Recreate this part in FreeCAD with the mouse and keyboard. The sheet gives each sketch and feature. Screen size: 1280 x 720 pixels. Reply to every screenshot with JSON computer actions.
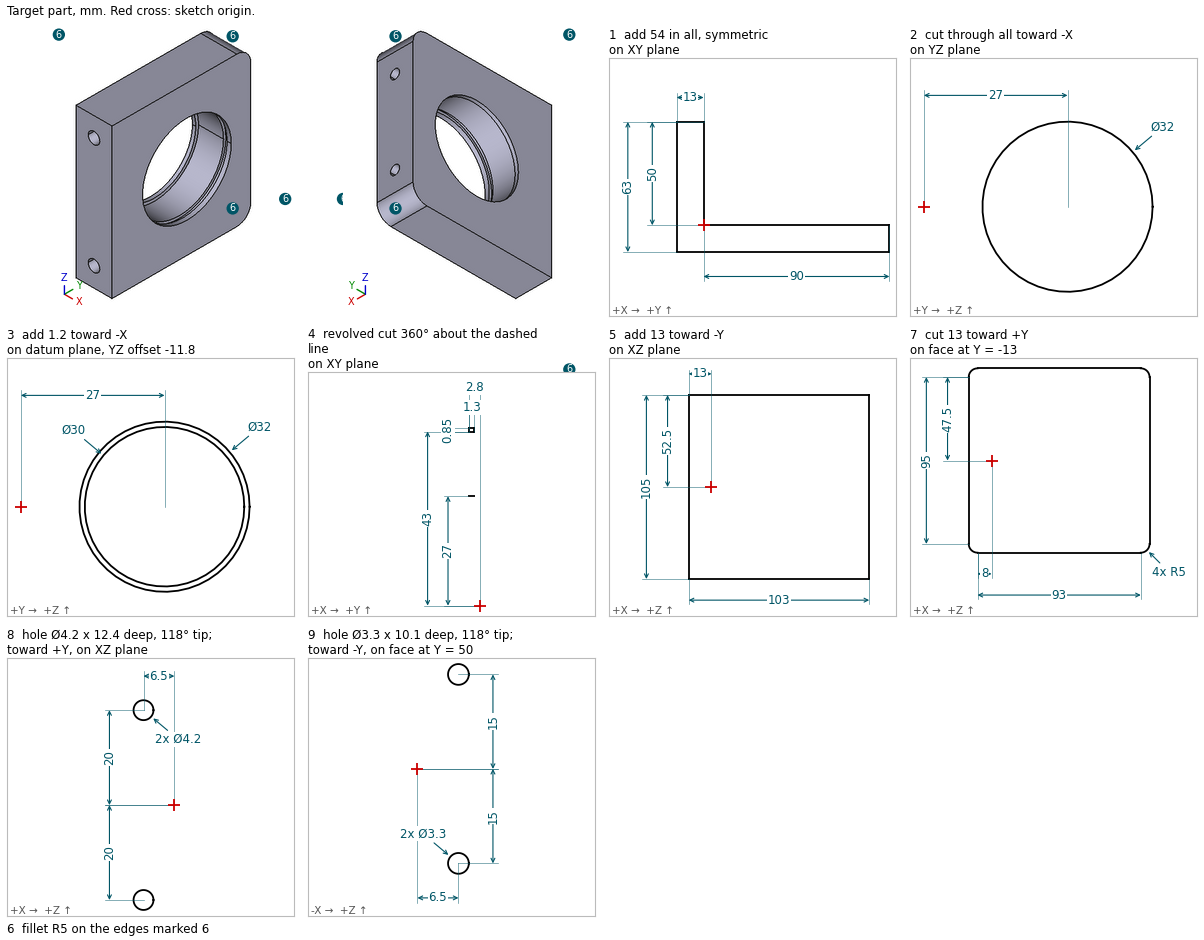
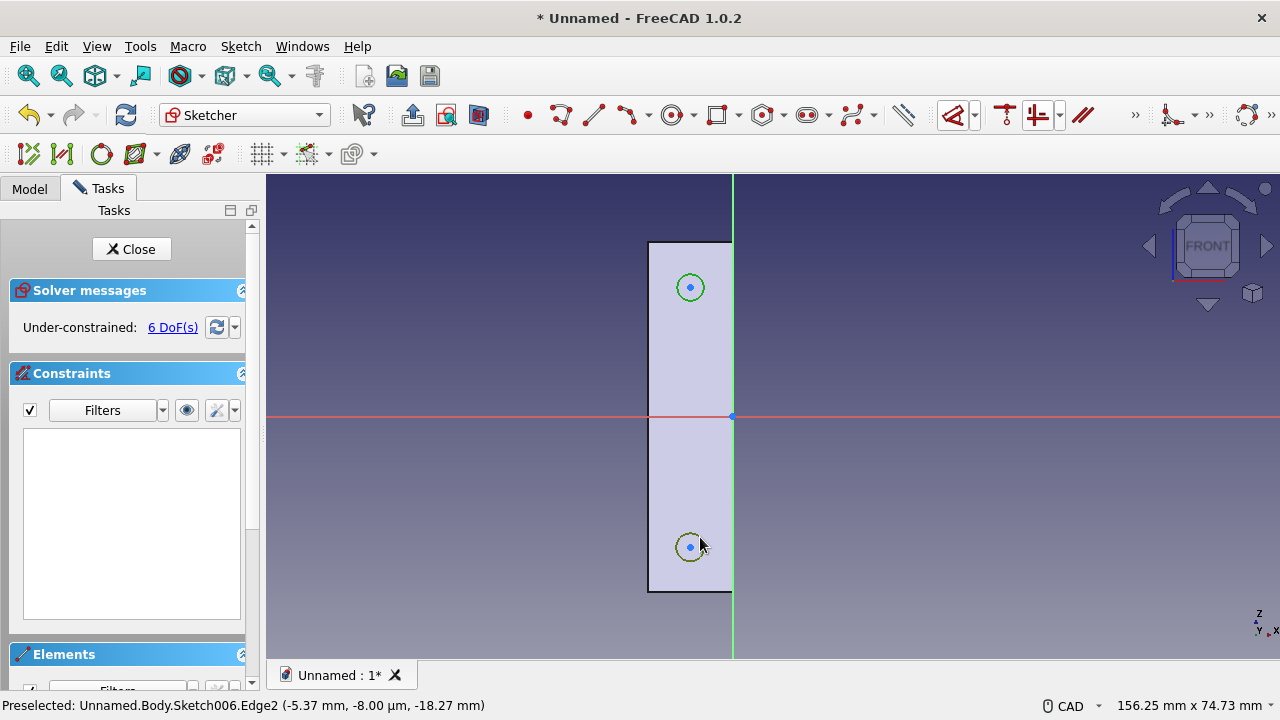
{"action": "key", "text": "e"}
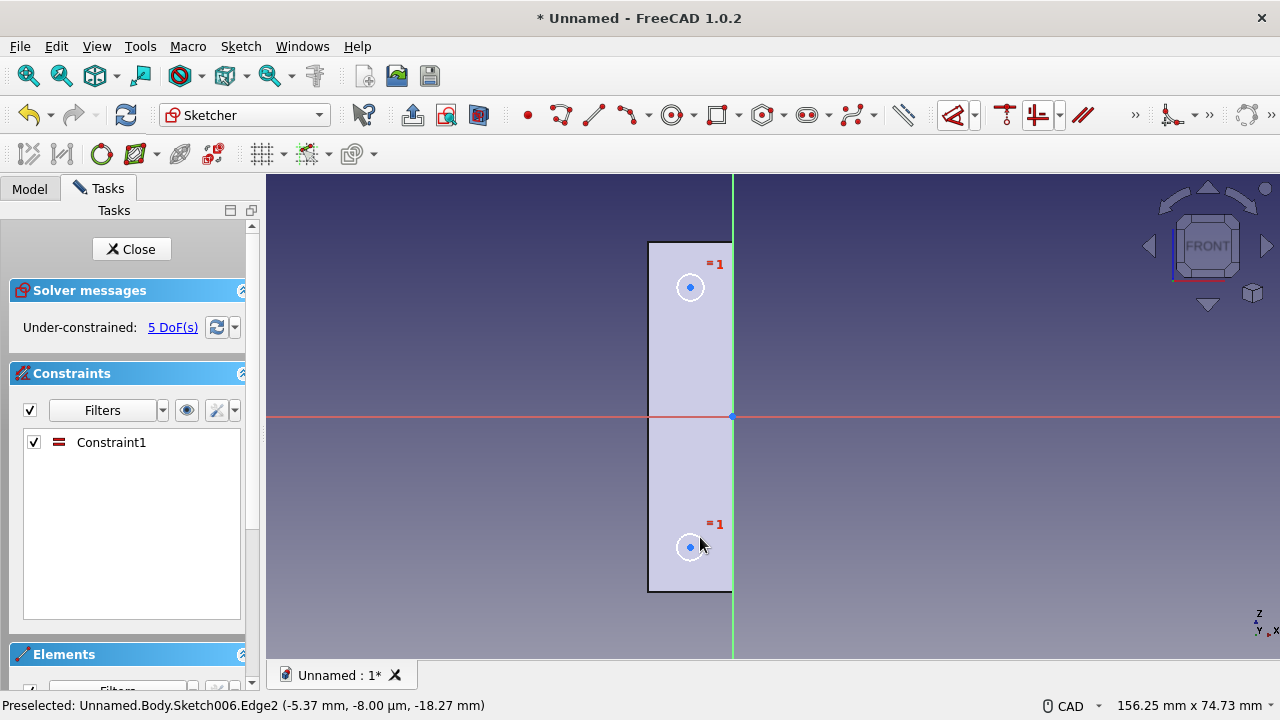
{"action": "left_click", "coordinate": [691, 288]}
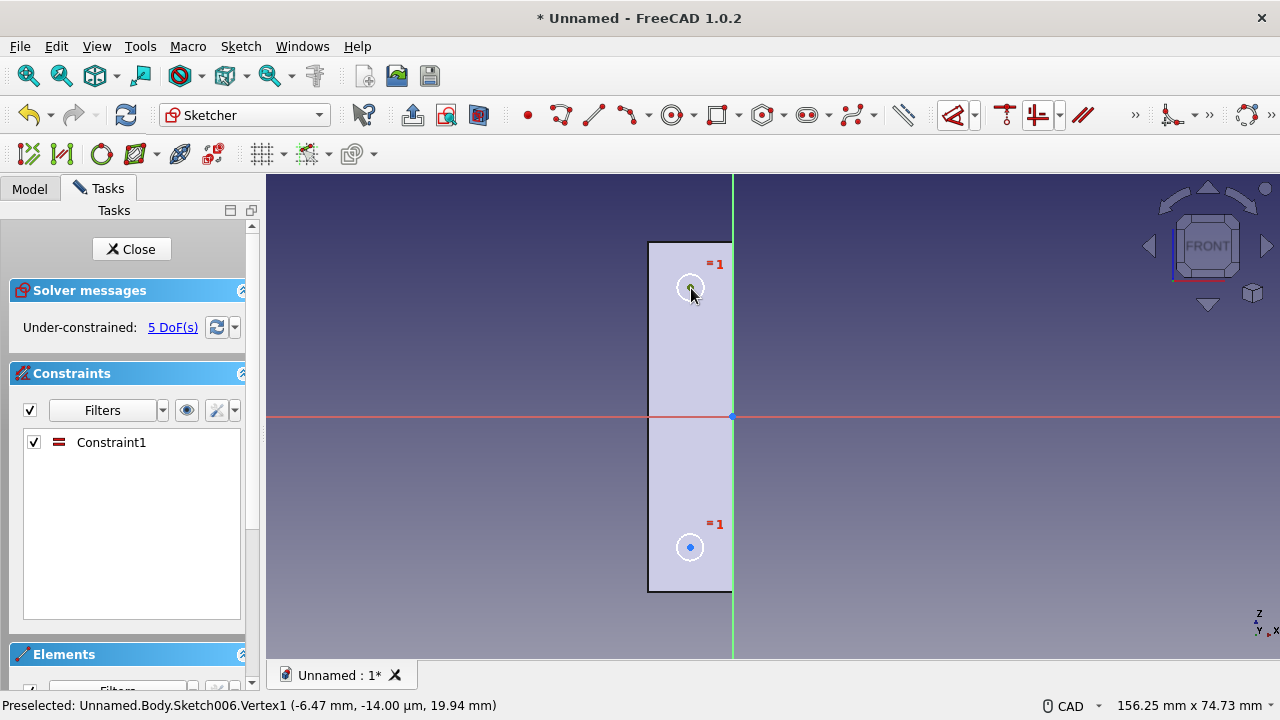
{"action": "left_click", "coordinate": [690, 547]}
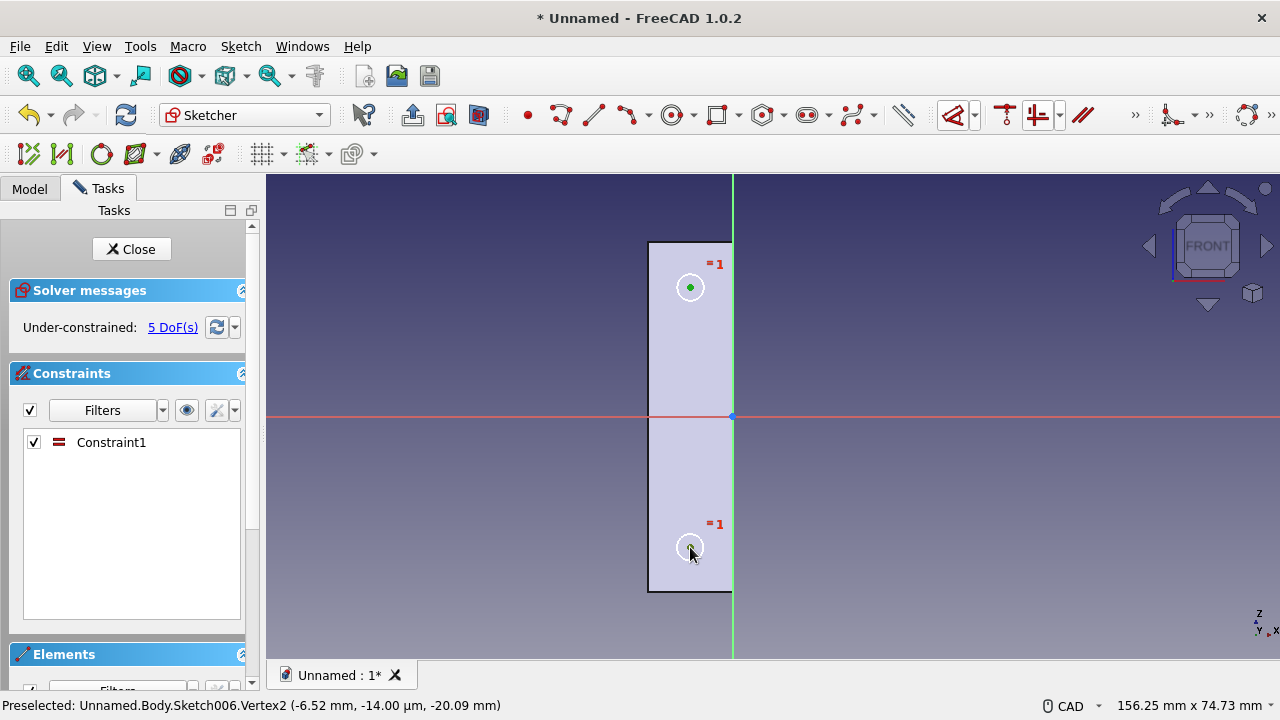
{"action": "key", "text": "v"}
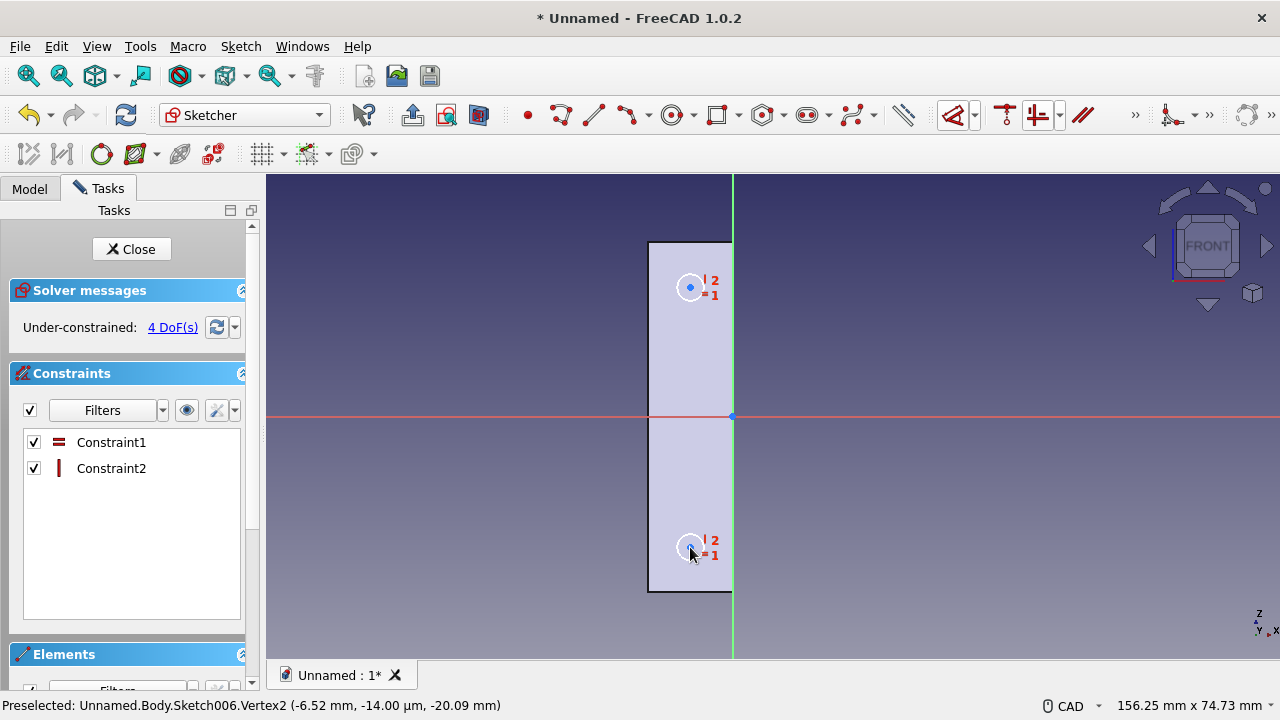
{"action": "scroll", "coordinate": [700, 278], "scroll_direction": "up", "scroll_amount": 2}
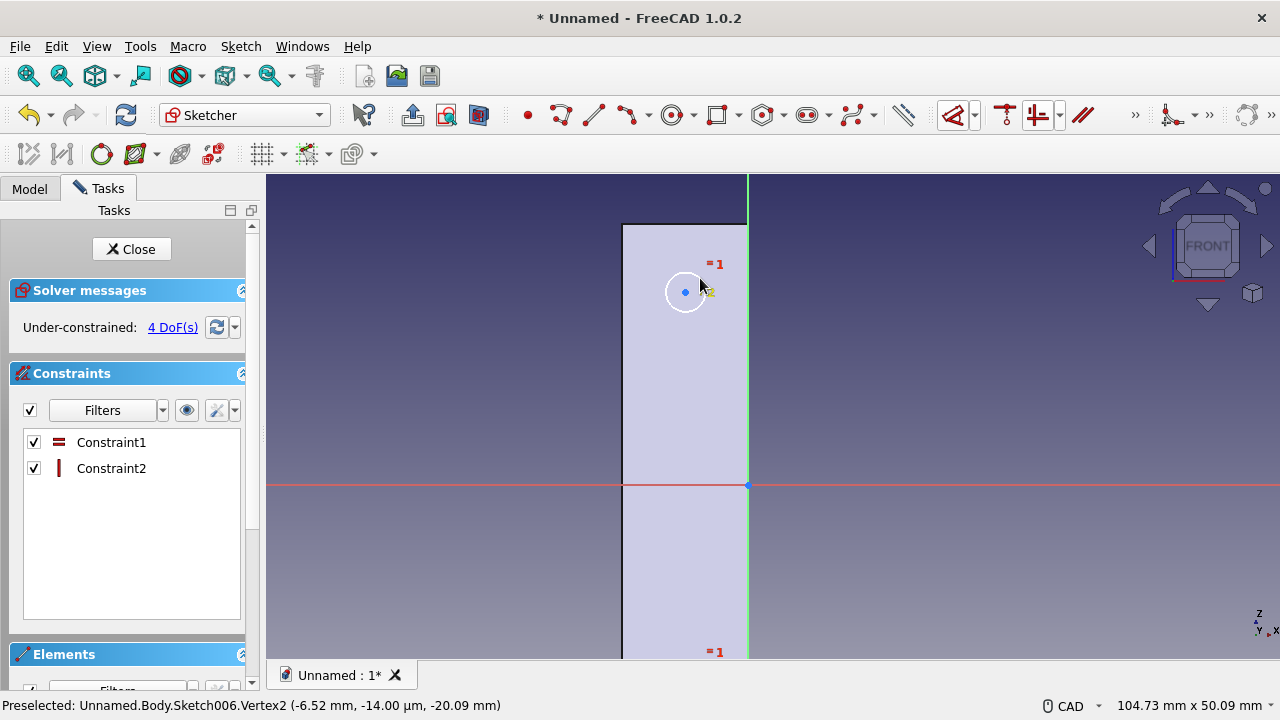
{"action": "left_click", "coordinate": [700, 278]}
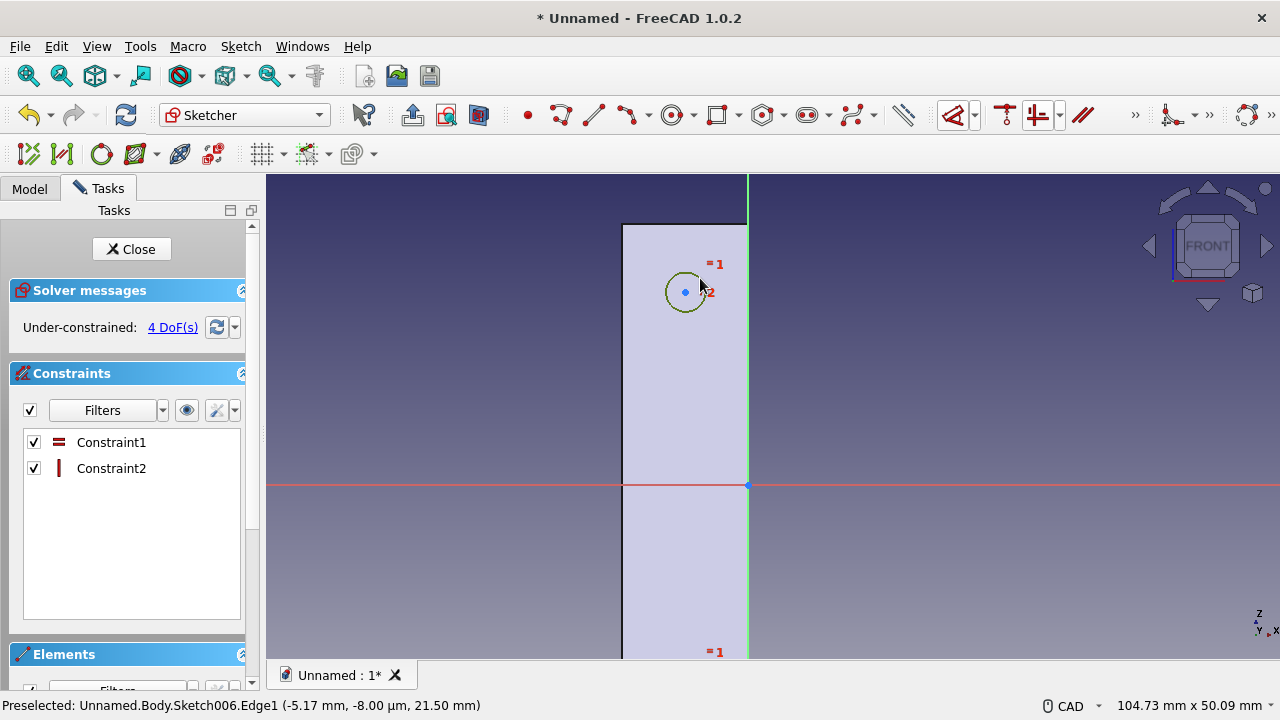
{"action": "left_click", "coordinate": [974, 116]}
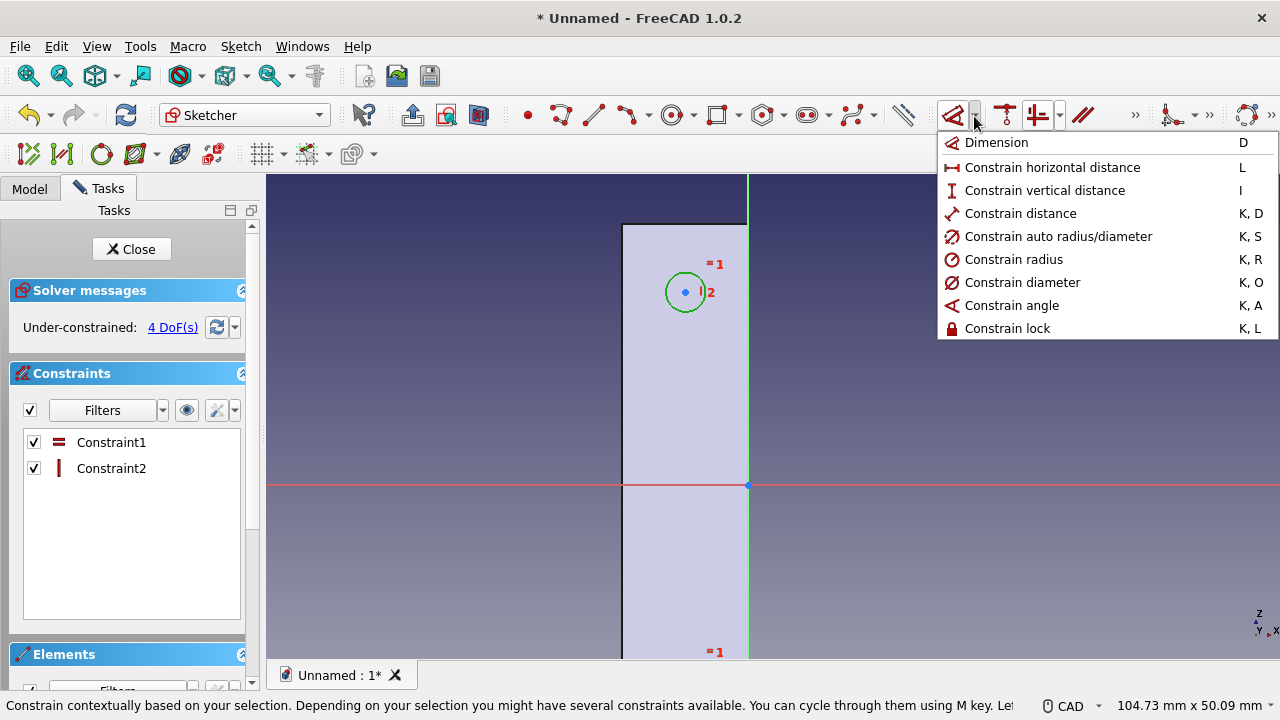
{"action": "left_click", "coordinate": [1108, 282]}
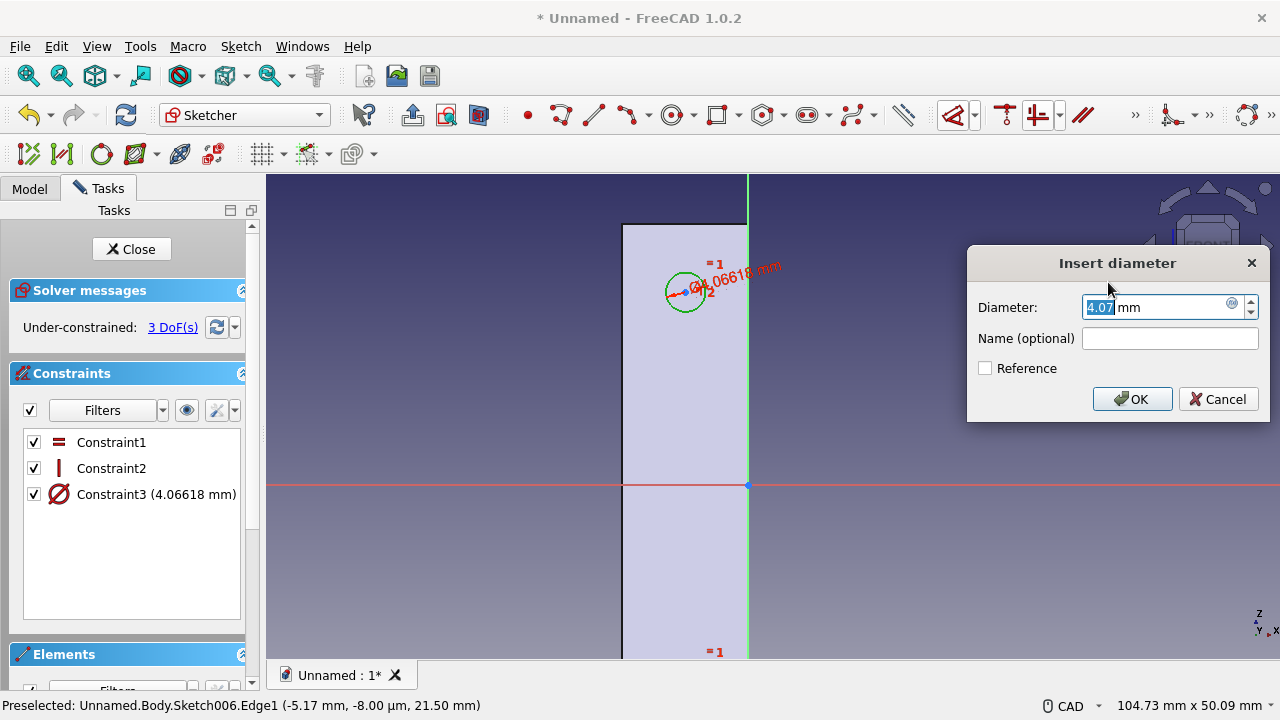
{"action": "type", "text": "4.2"}
{"action": "key", "text": "Return"}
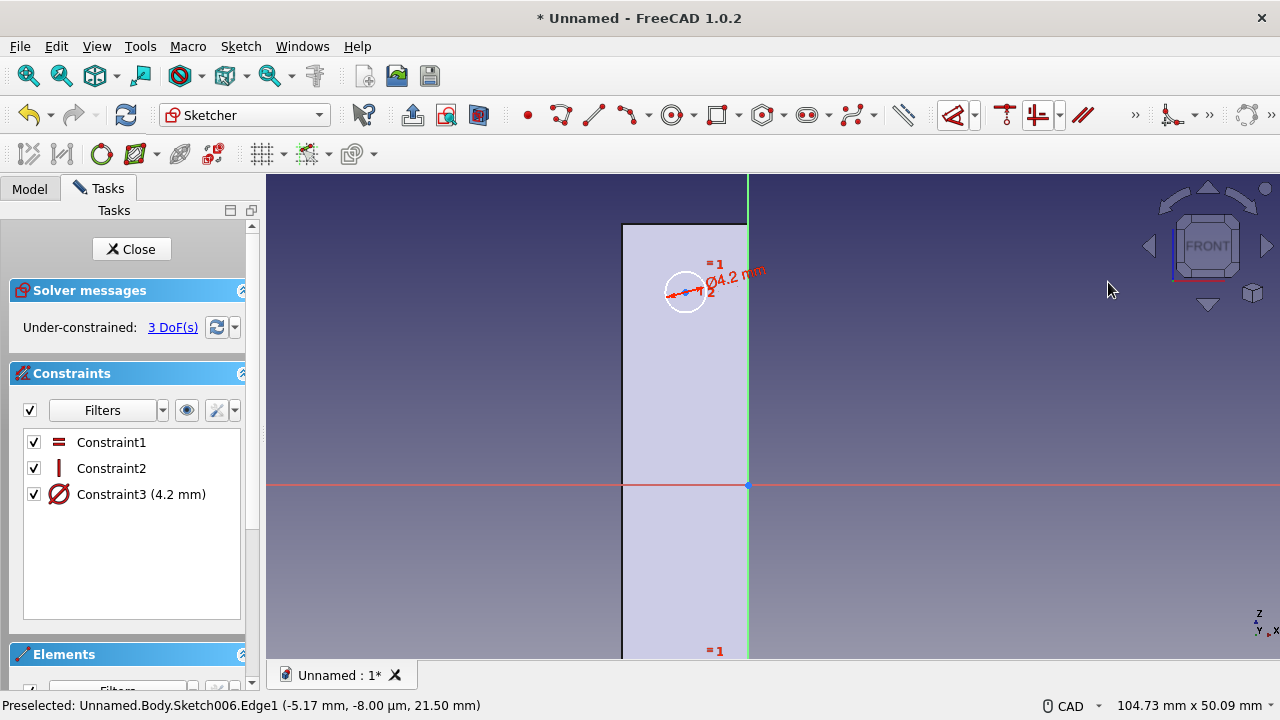
{"action": "left_click", "coordinate": [686, 292]}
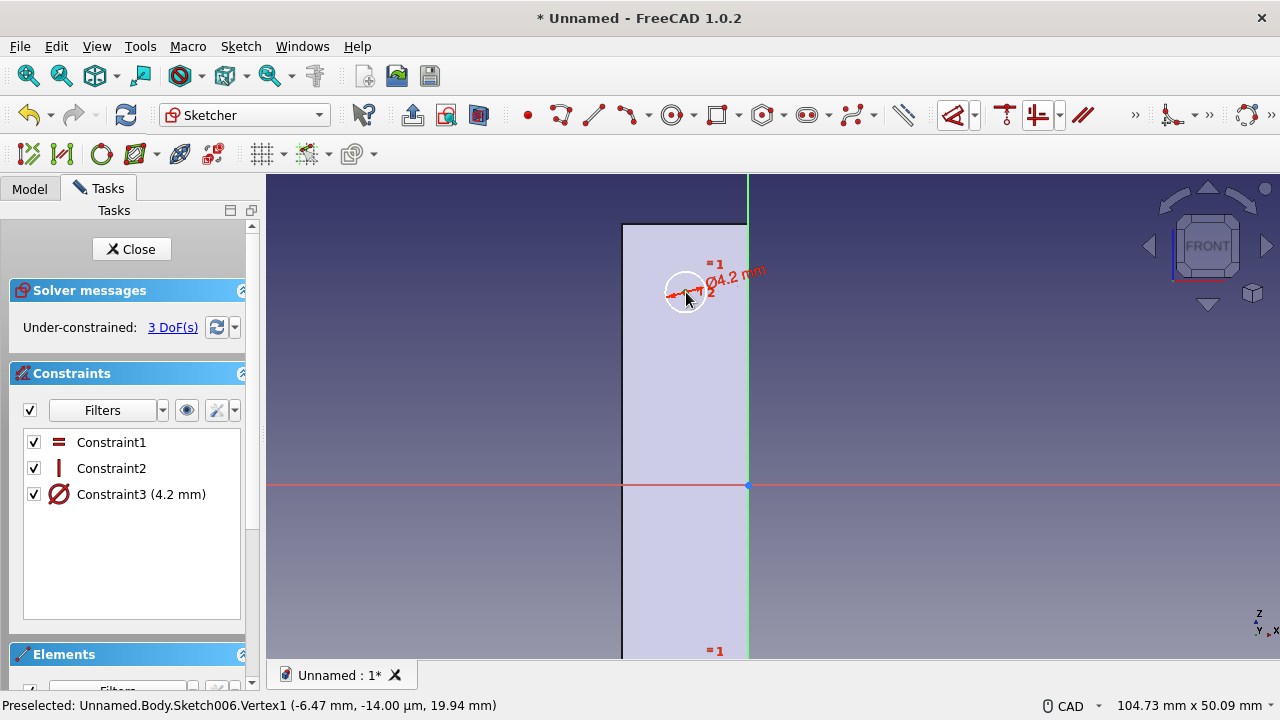
{"action": "left_click", "coordinate": [974, 116]}